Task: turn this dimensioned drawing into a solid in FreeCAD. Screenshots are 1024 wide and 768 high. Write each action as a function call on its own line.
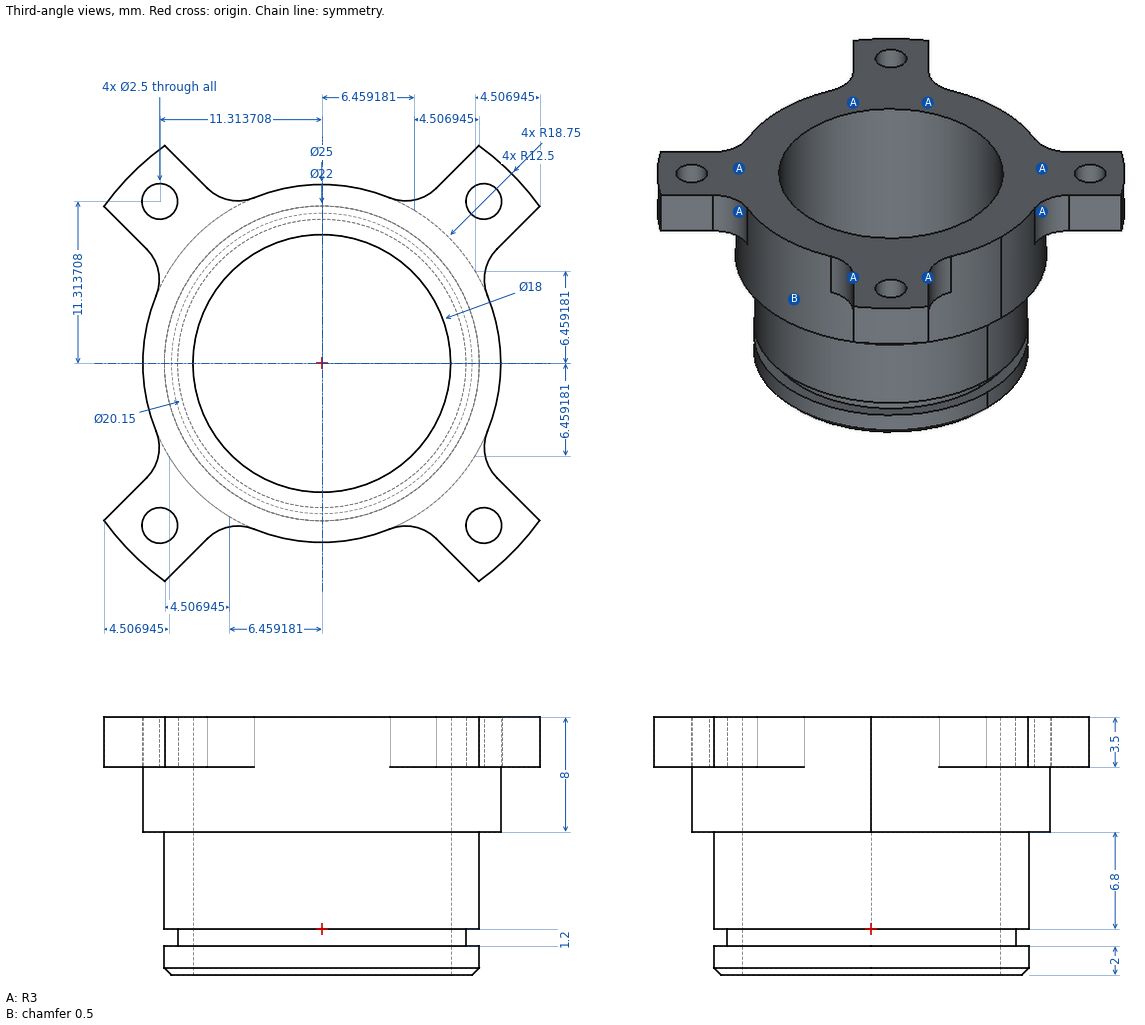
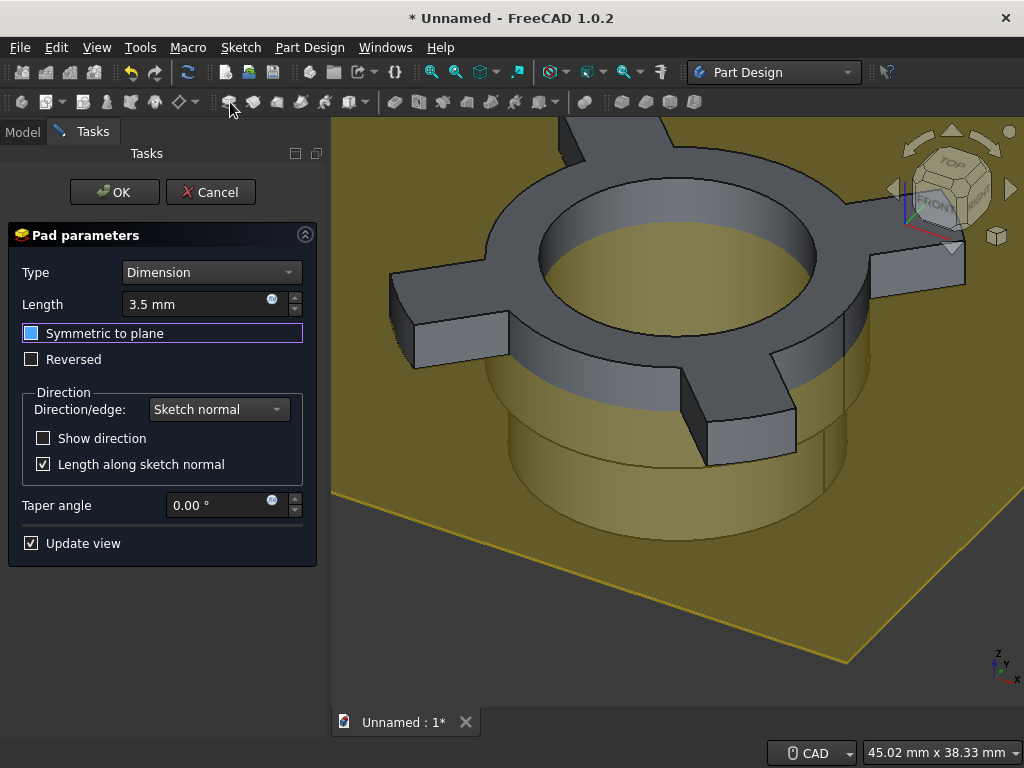
click(115, 192)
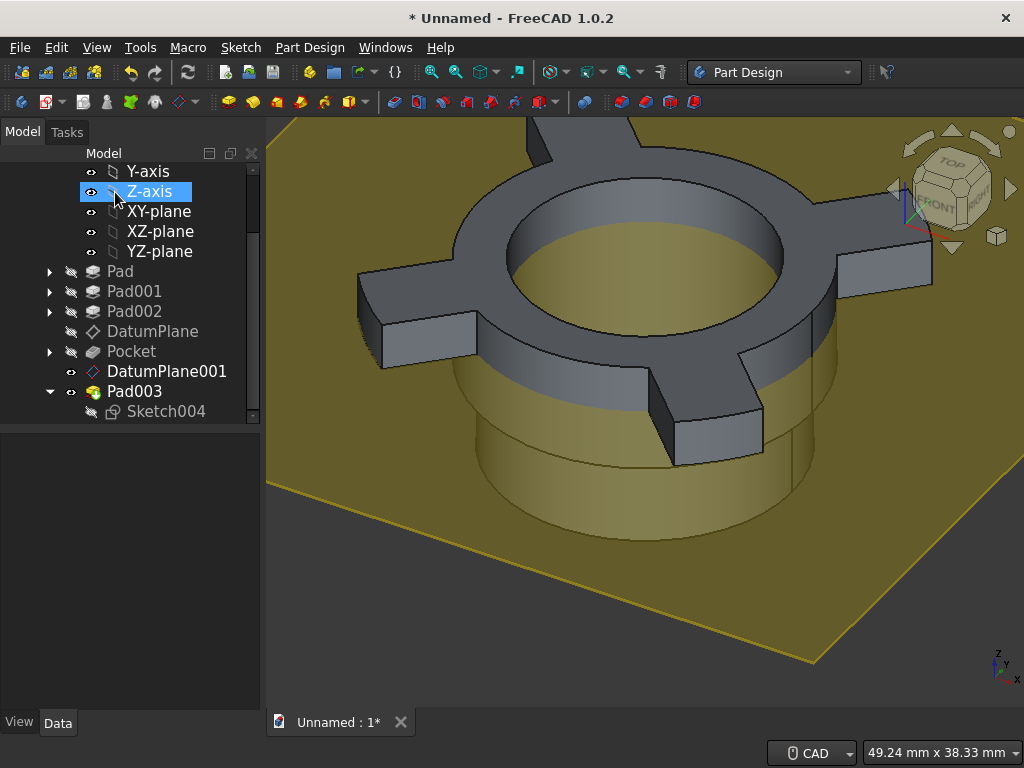
click(116, 372)
key(space)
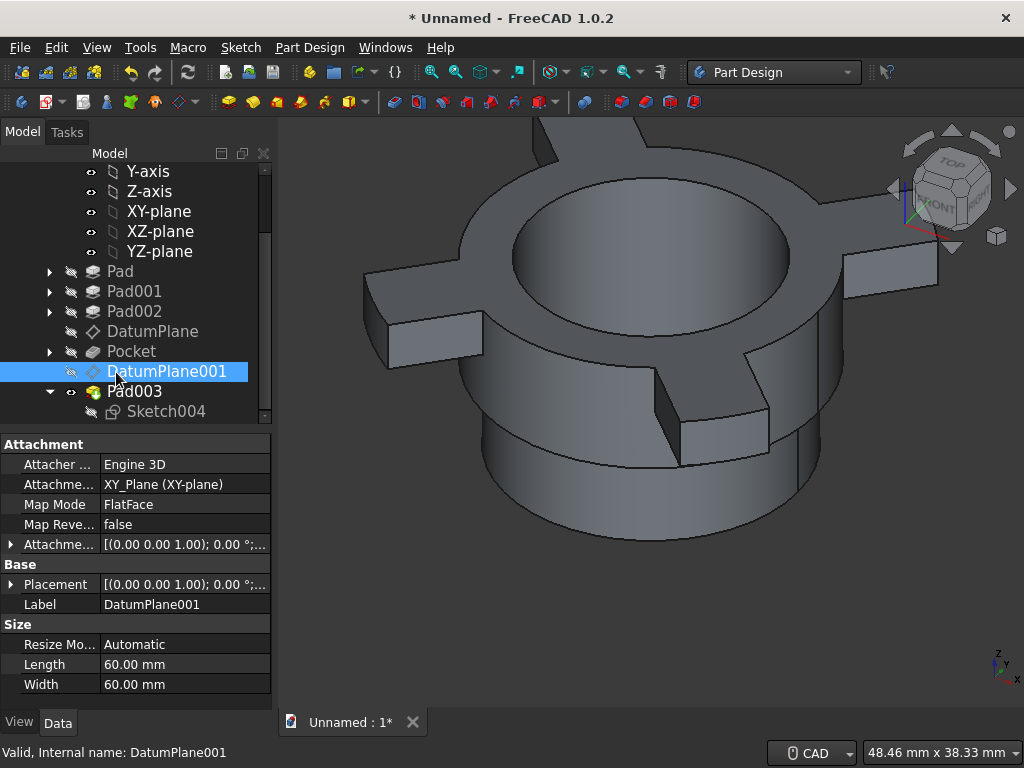
click(432, 72)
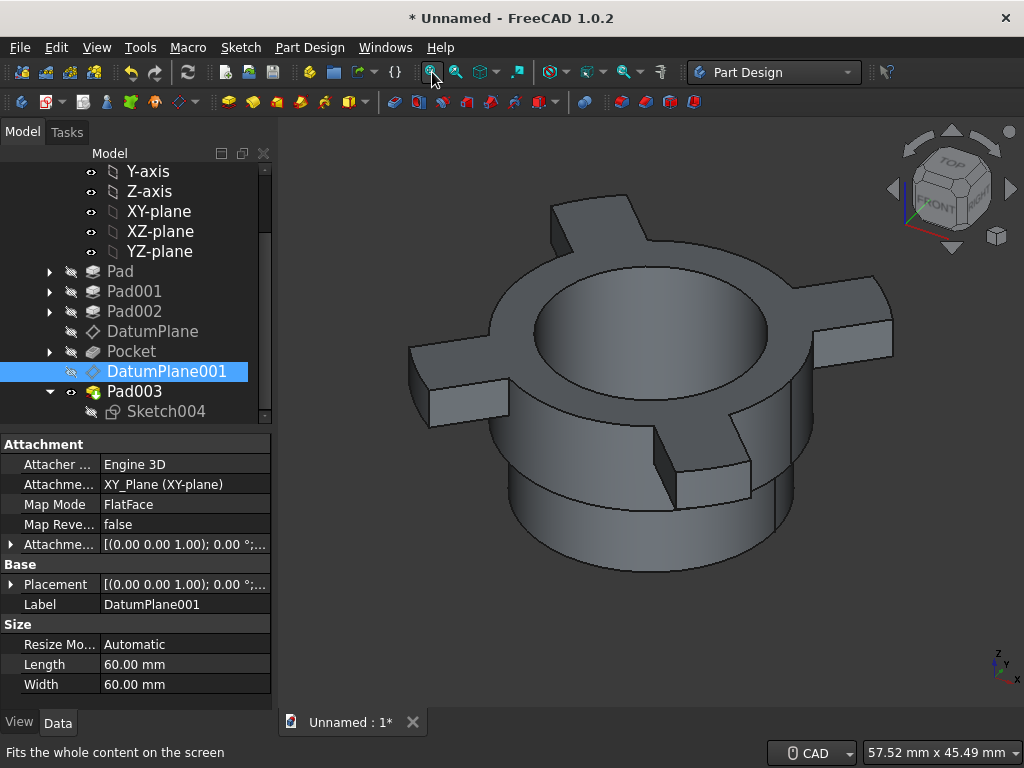
click(692, 421)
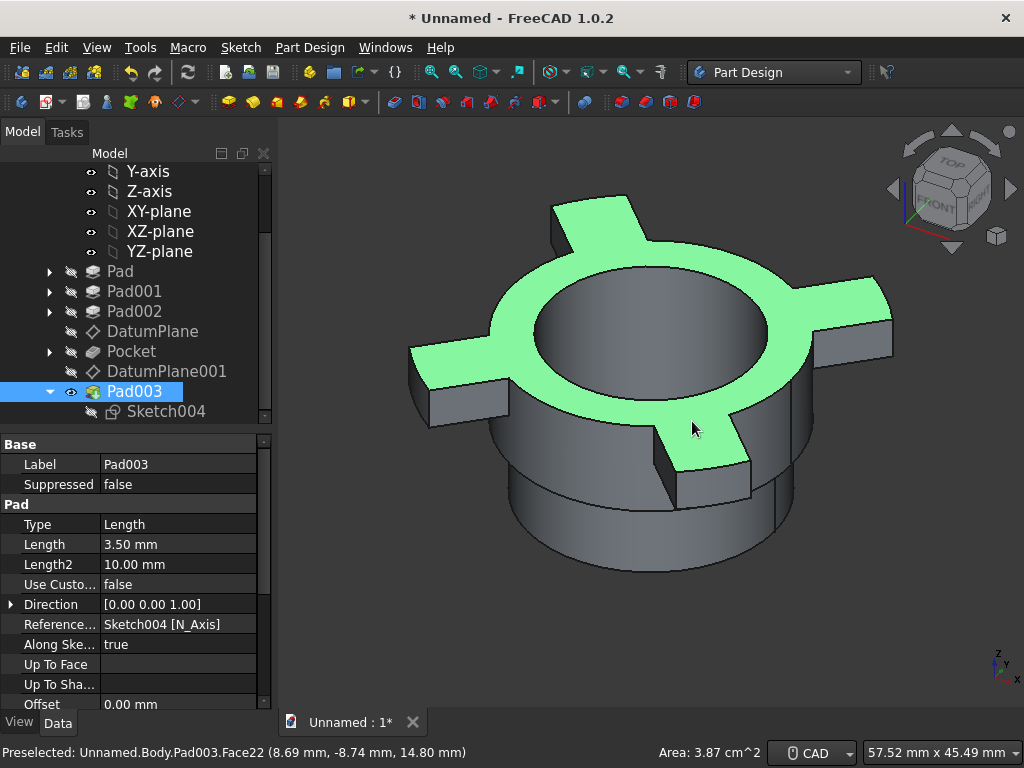
click(46, 102)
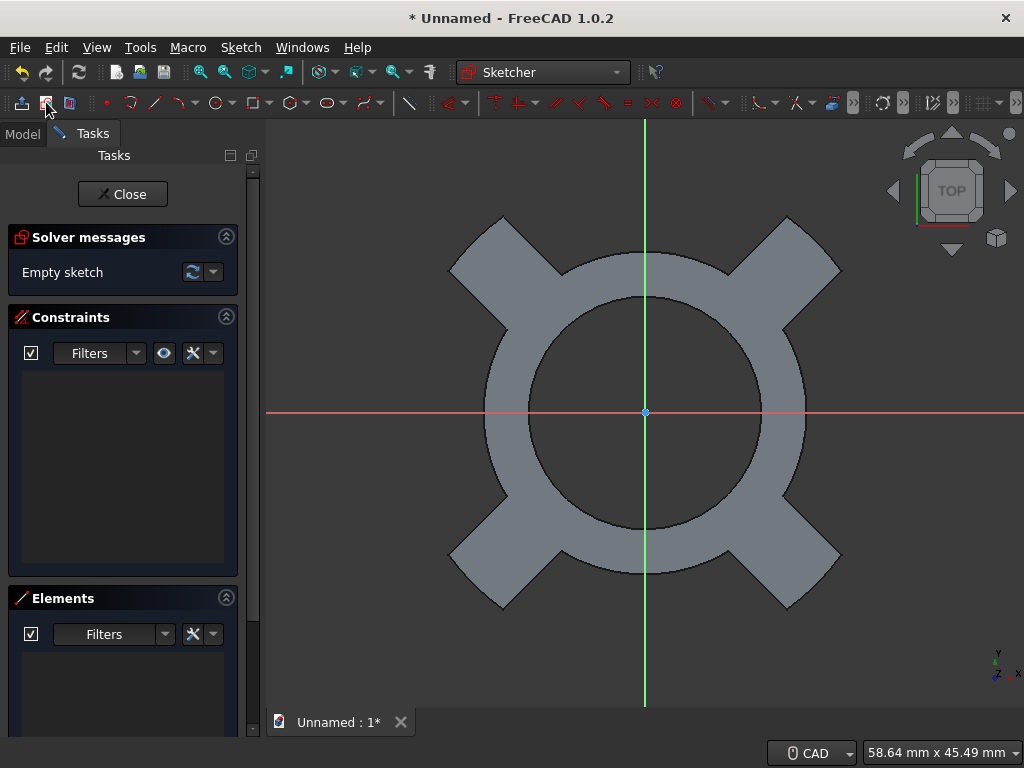
click(216, 104)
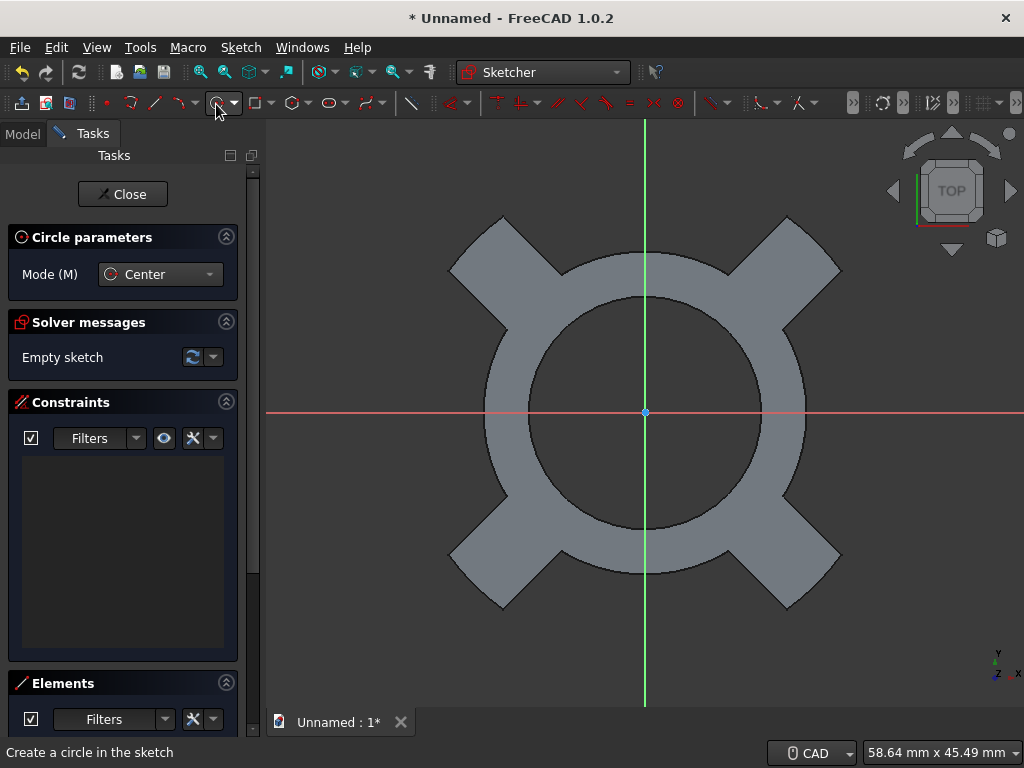
scroll(499, 267, up, 2)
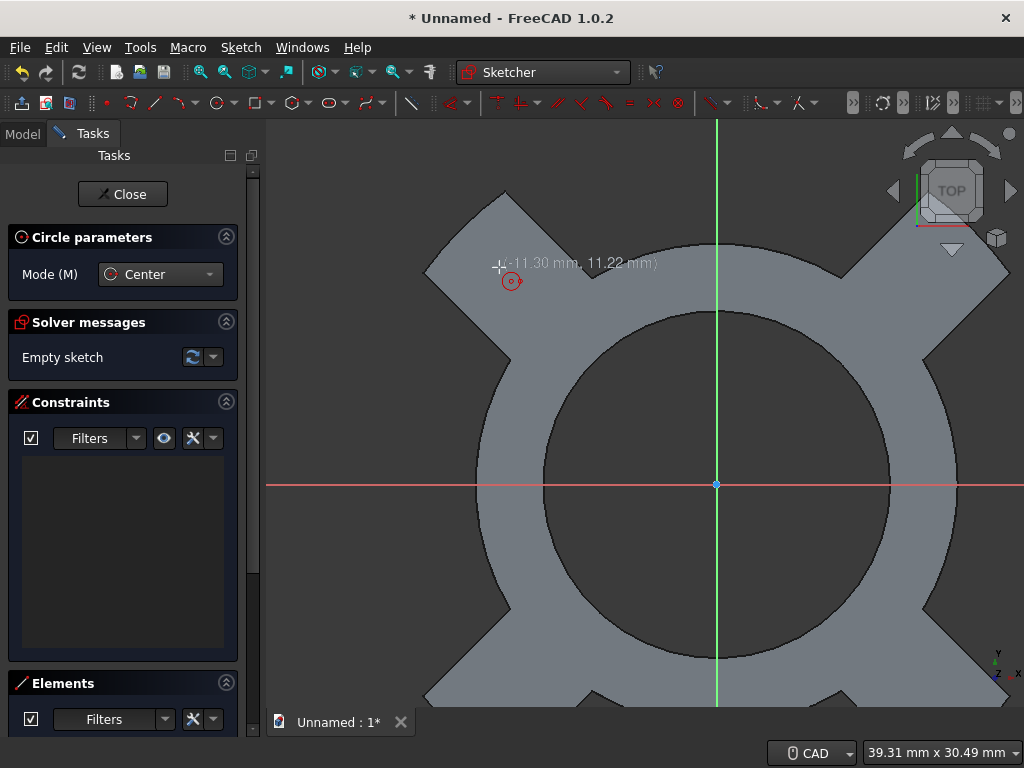
click(498, 267)
click(516, 249)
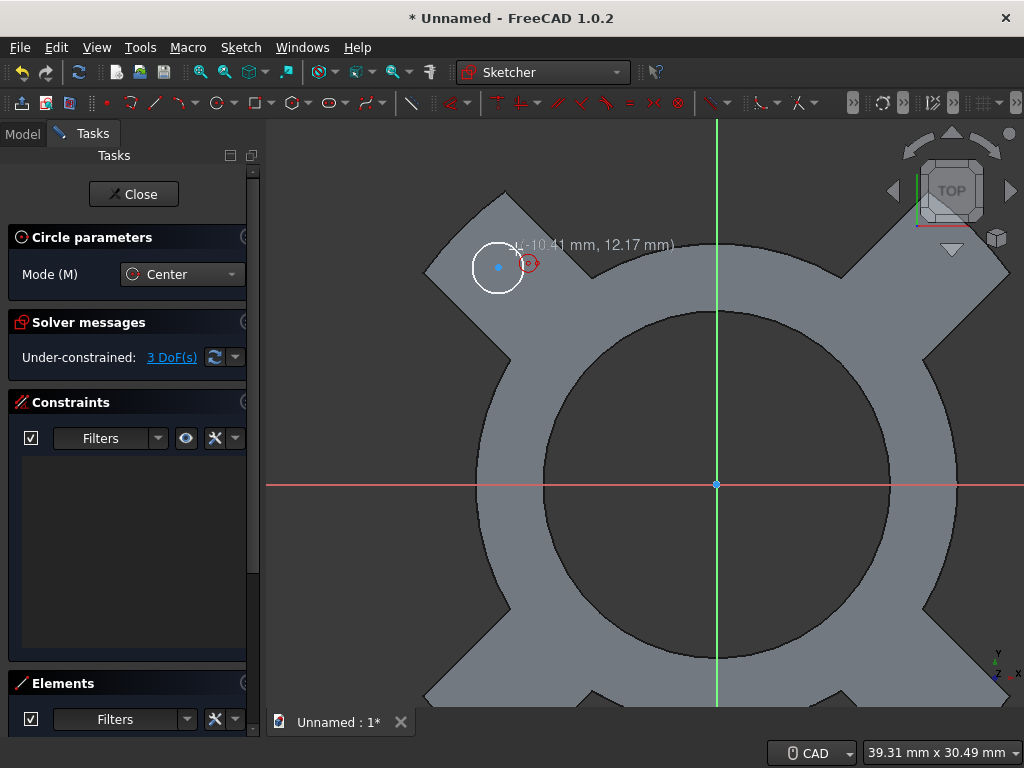
scroll(294, 267, down, 2)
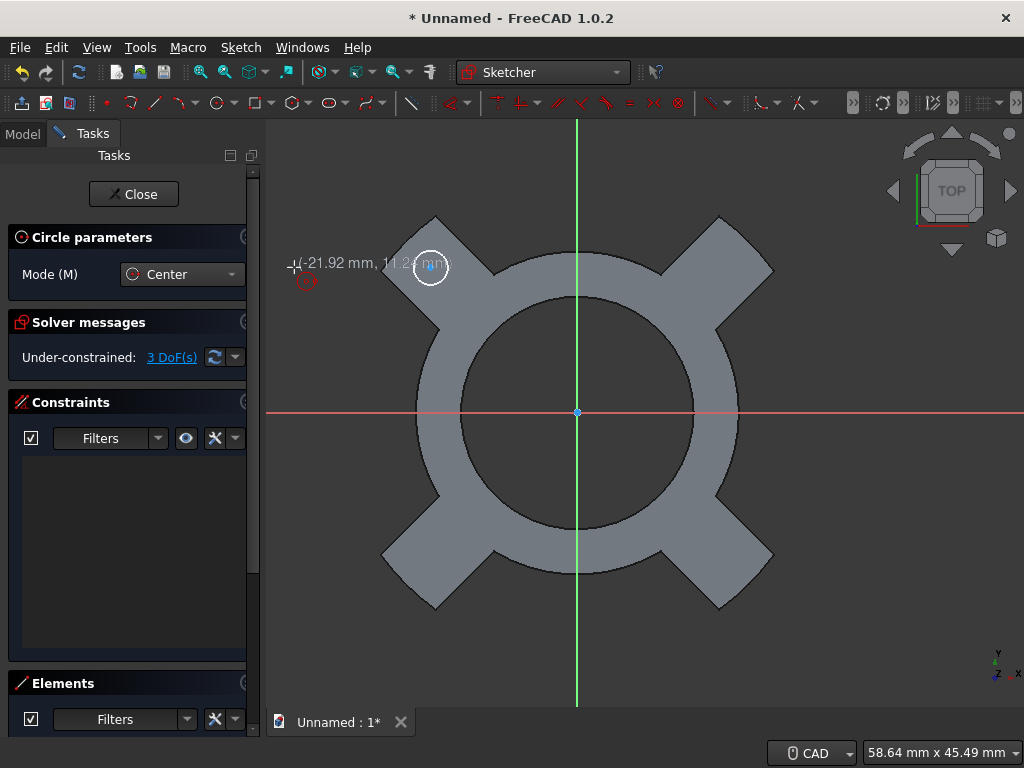
scroll(724, 267, up, 2)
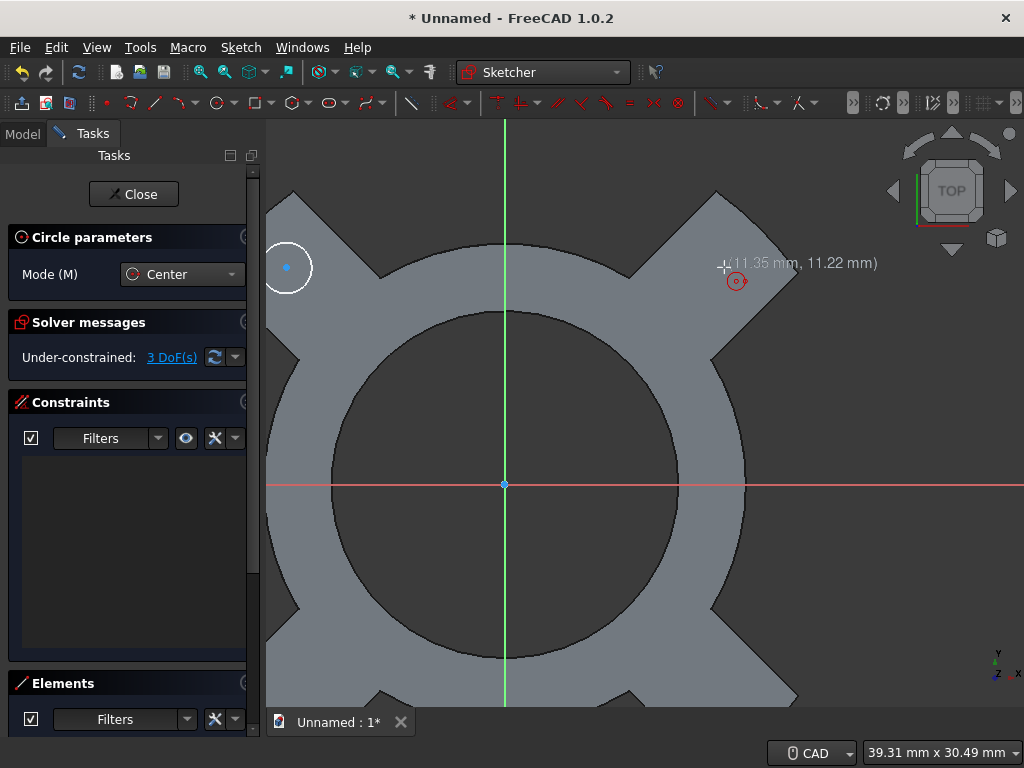
click(723, 267)
click(740, 249)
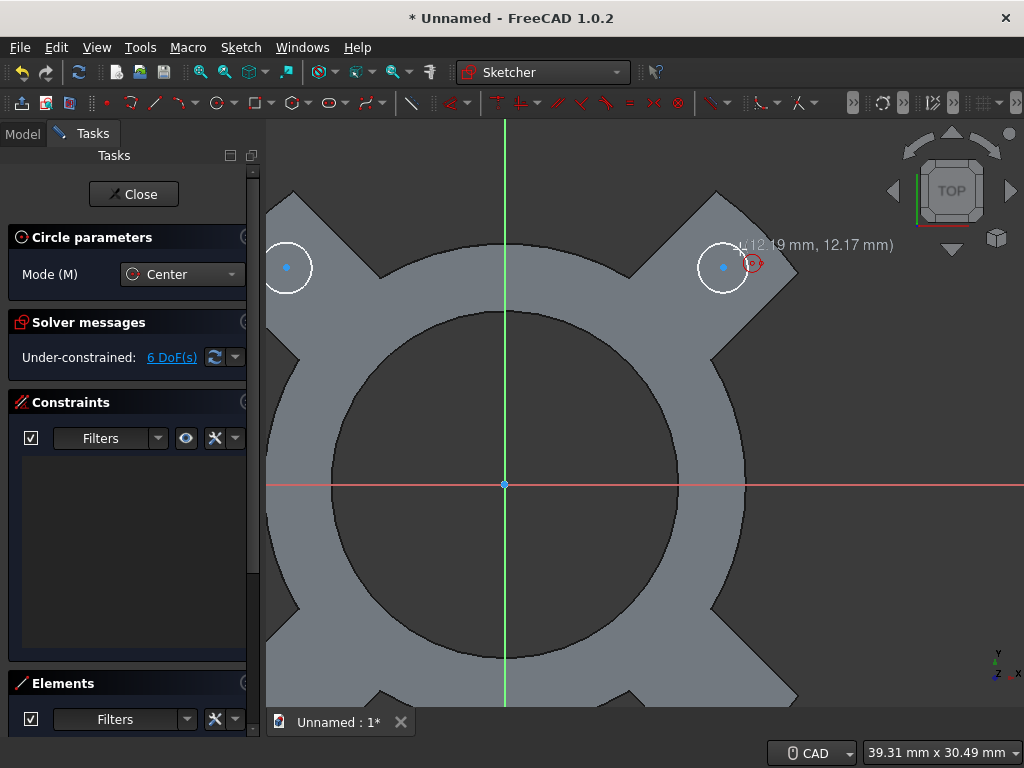
scroll(859, 147, down, 1)